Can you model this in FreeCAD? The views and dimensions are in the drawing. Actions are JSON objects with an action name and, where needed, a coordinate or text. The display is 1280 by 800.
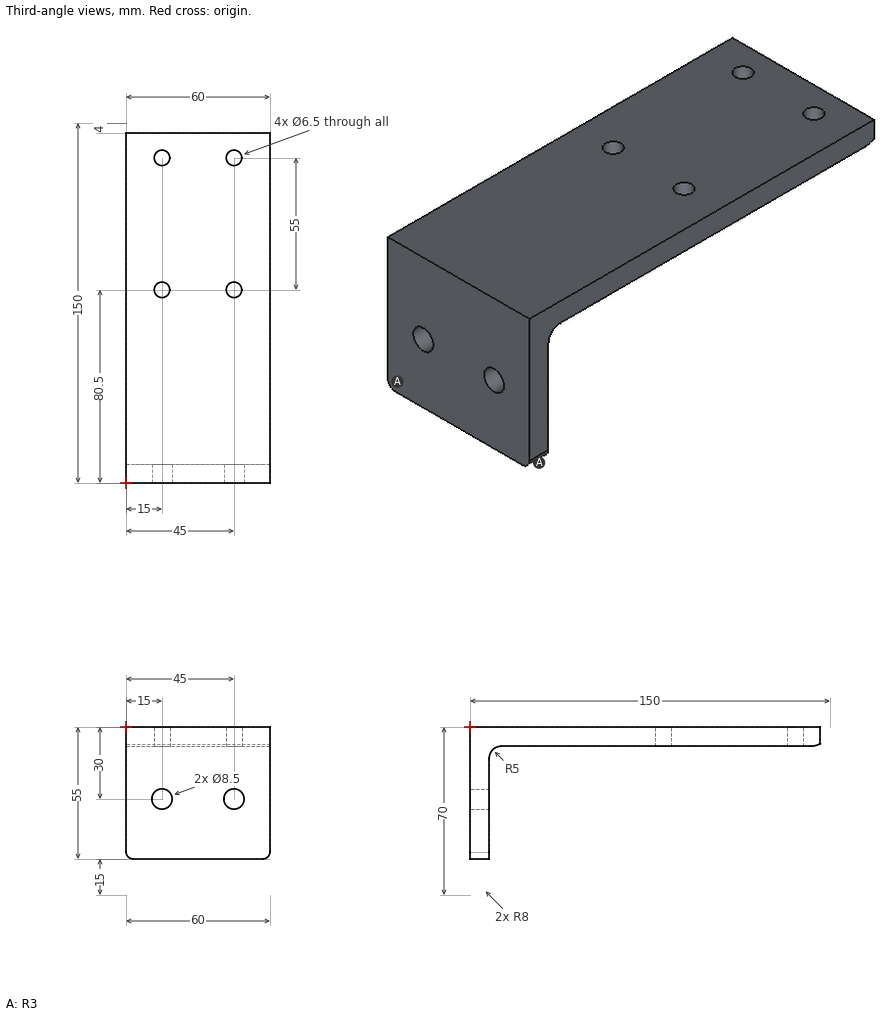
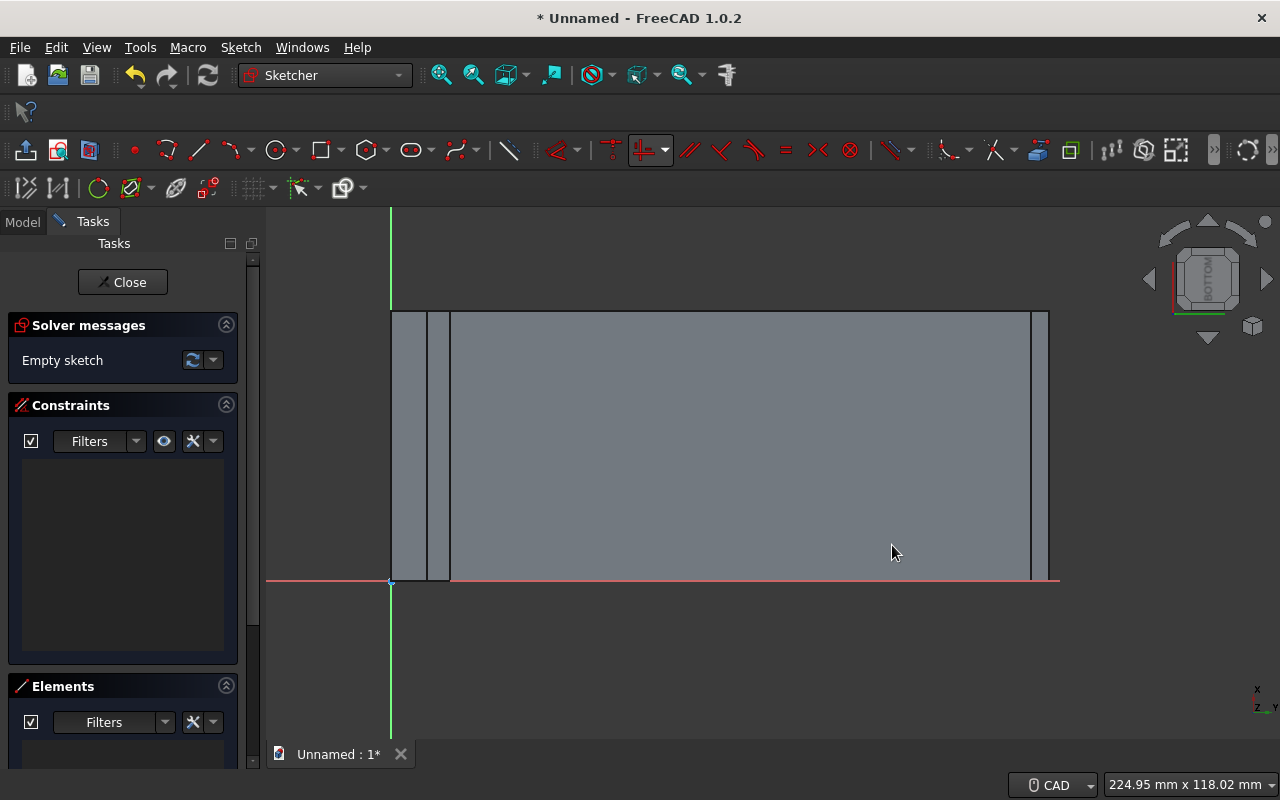
{"action": "left_click", "coordinate": [276, 150]}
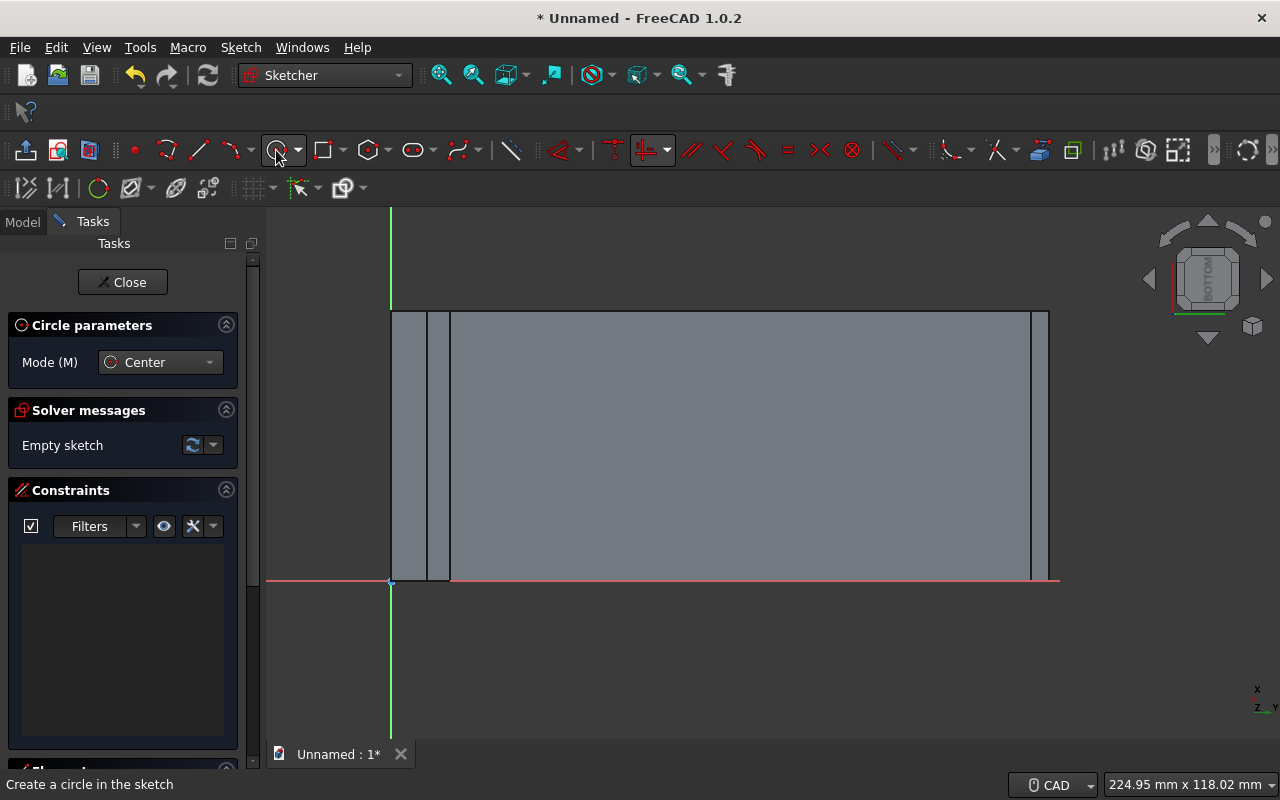
{"action": "scroll", "coordinate": [1002, 379], "scroll_direction": "up", "scroll_amount": 3}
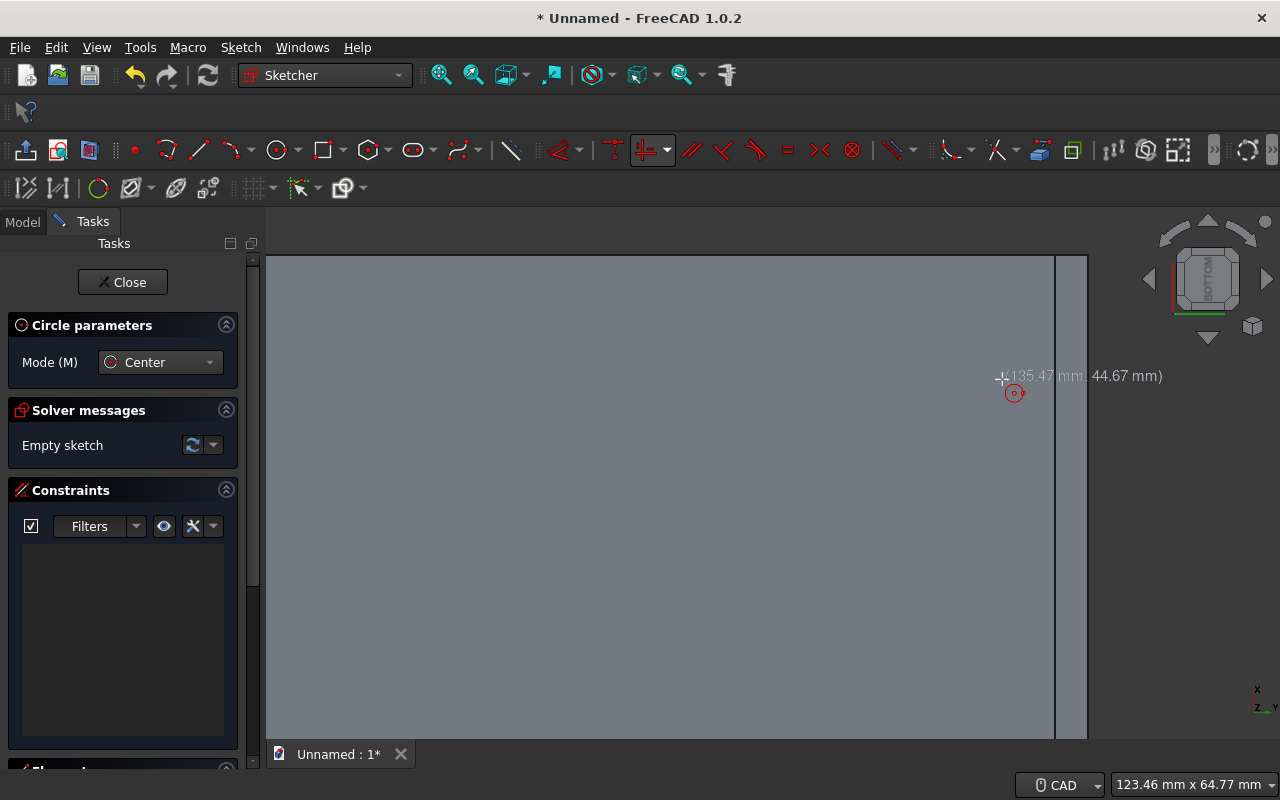
{"action": "left_click", "coordinate": [1002, 378]}
{"action": "left_click", "coordinate": [1021, 359]}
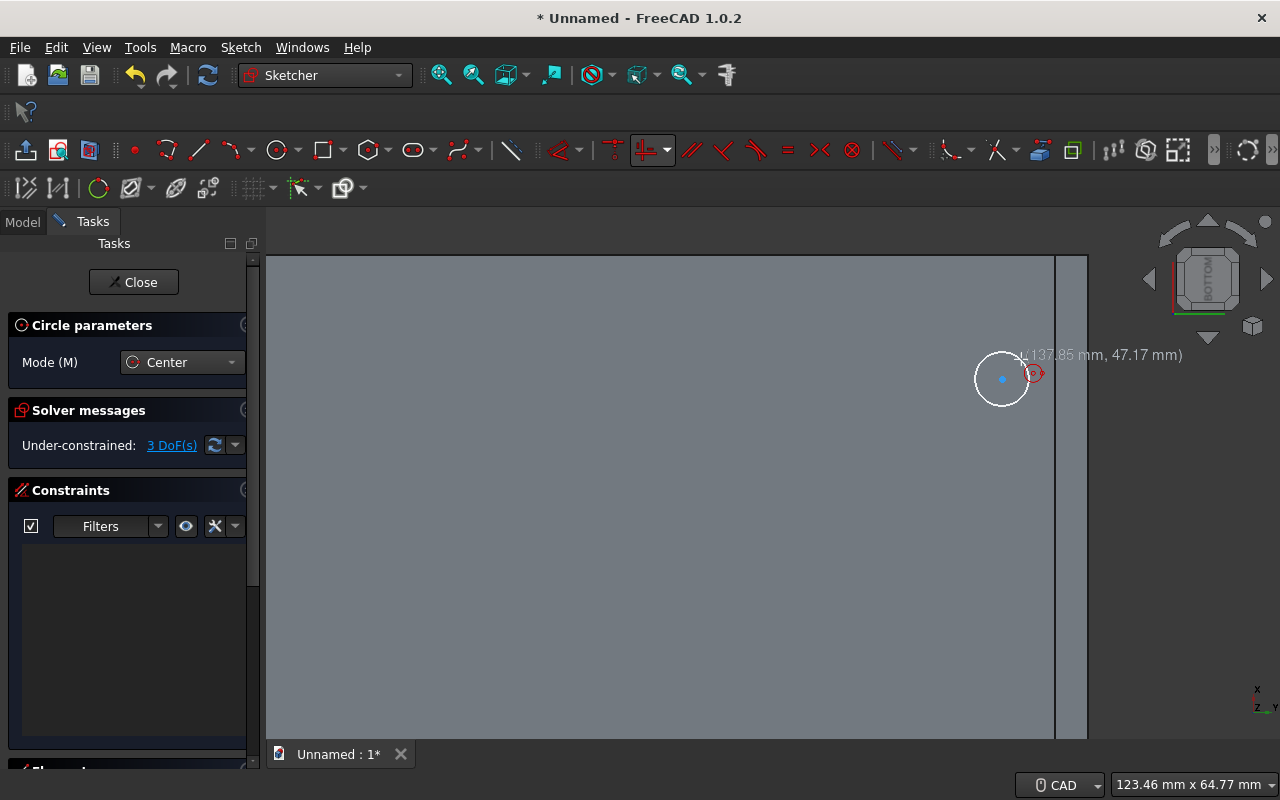
{"action": "left_click", "coordinate": [1002, 624]}
{"action": "left_click", "coordinate": [1021, 605]}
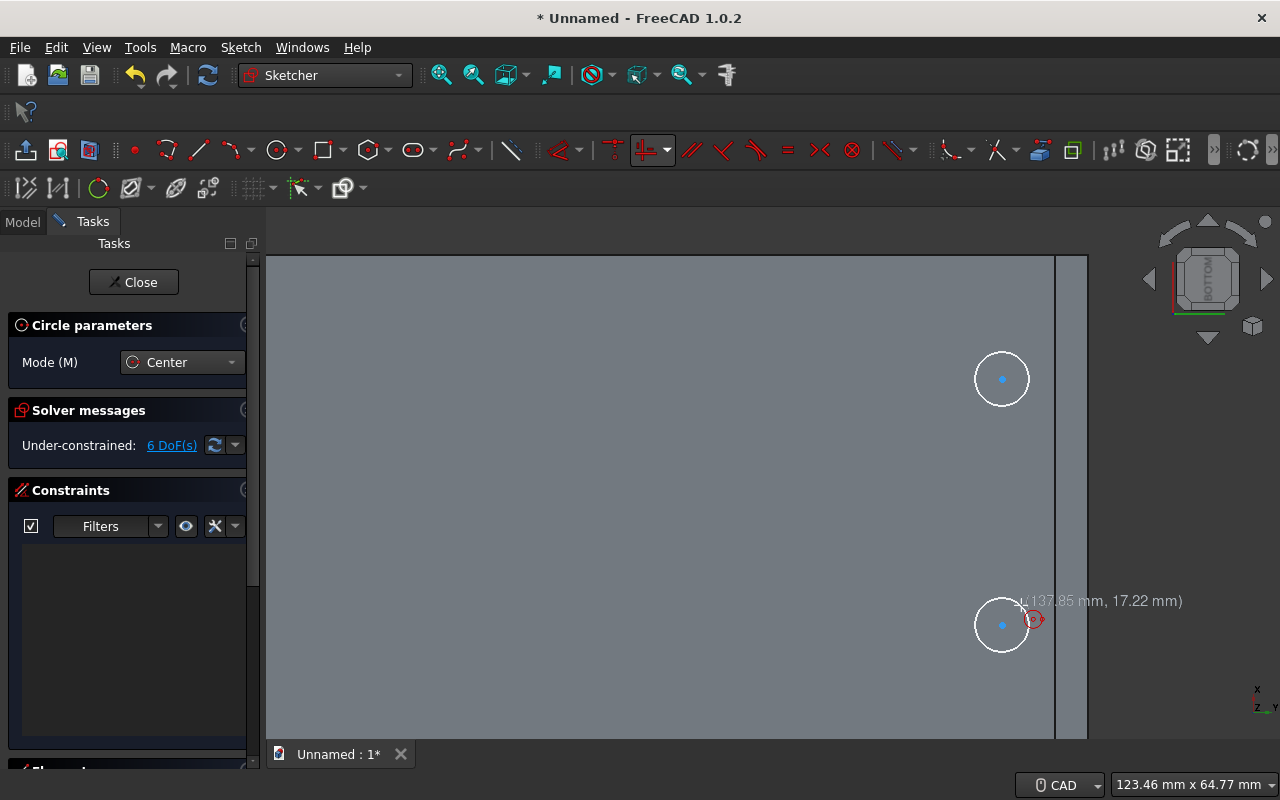
{"action": "left_click", "coordinate": [550, 378]}
{"action": "left_click", "coordinate": [569, 359]}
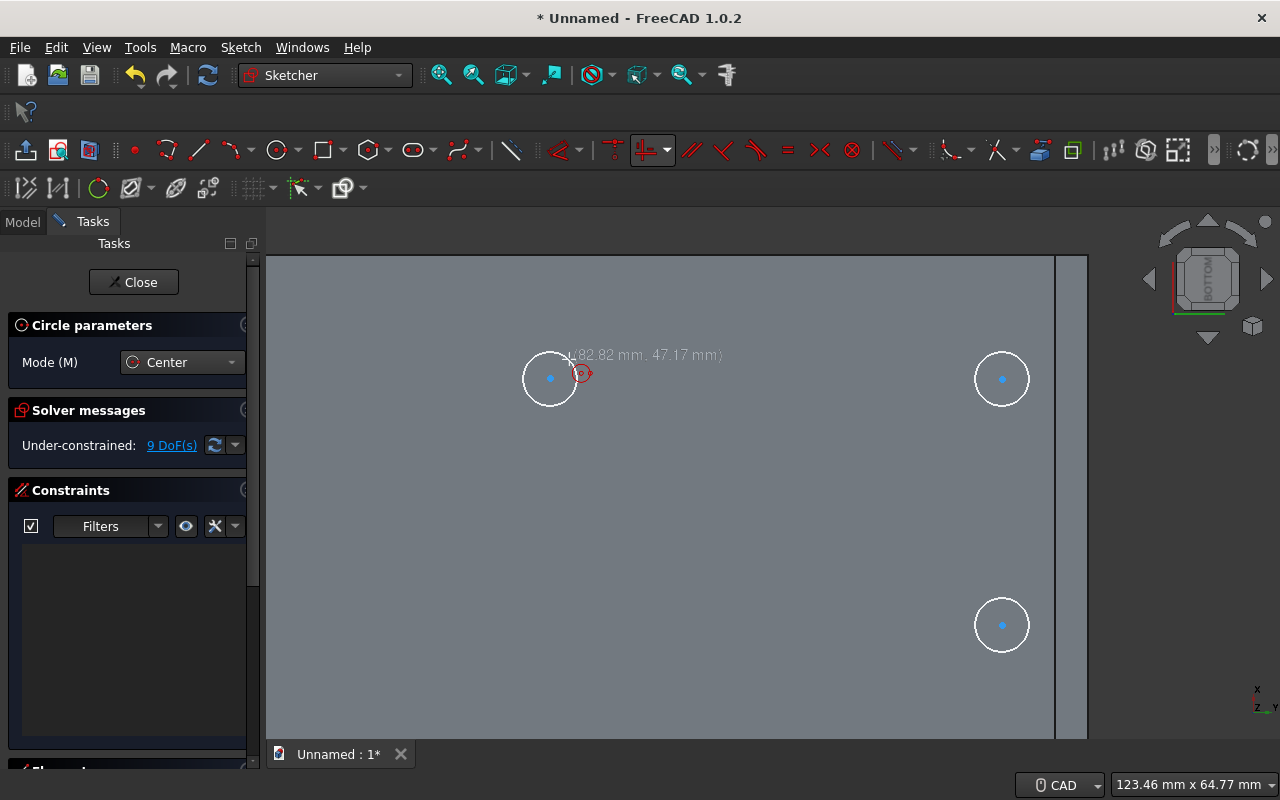
{"action": "left_click", "coordinate": [550, 624]}
{"action": "left_click", "coordinate": [569, 605]}
{"action": "key", "text": "Escape"}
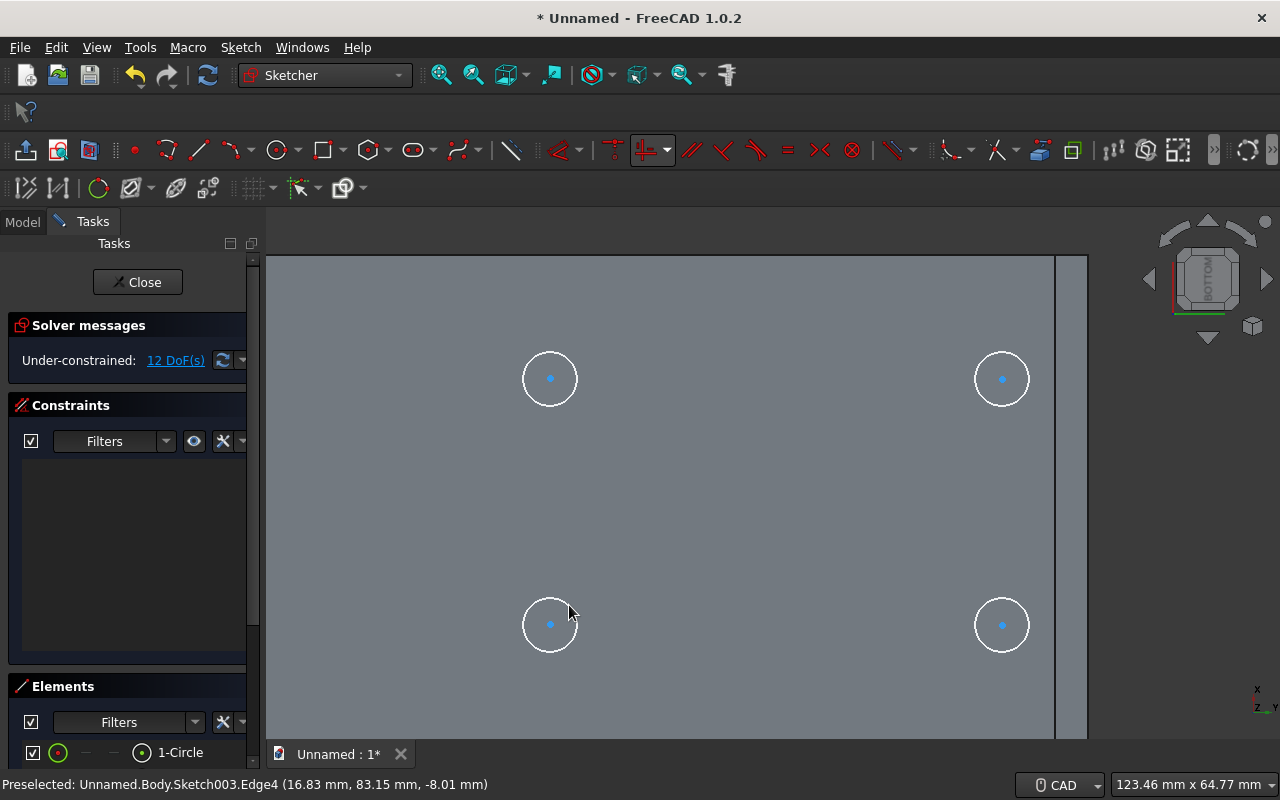
{"action": "left_click", "coordinate": [1021, 360]}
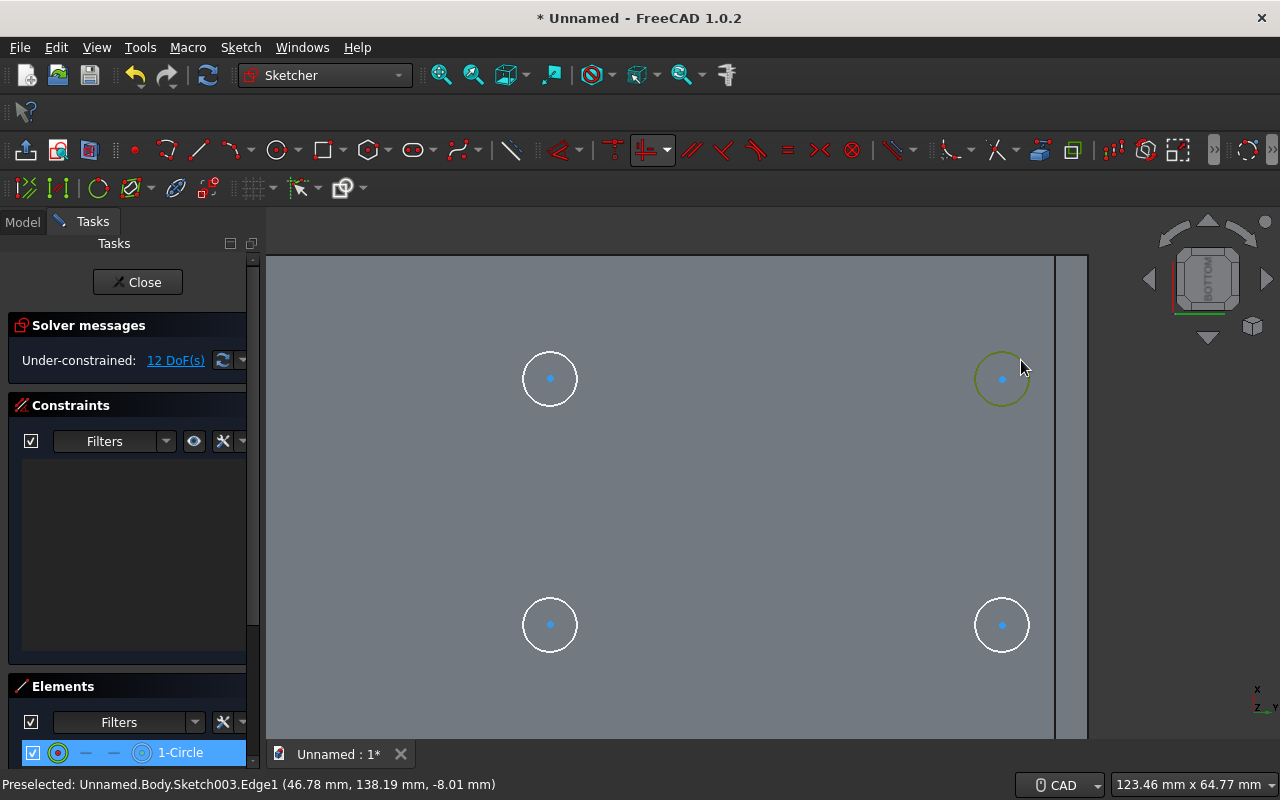
{"action": "left_click", "coordinate": [1021, 606]}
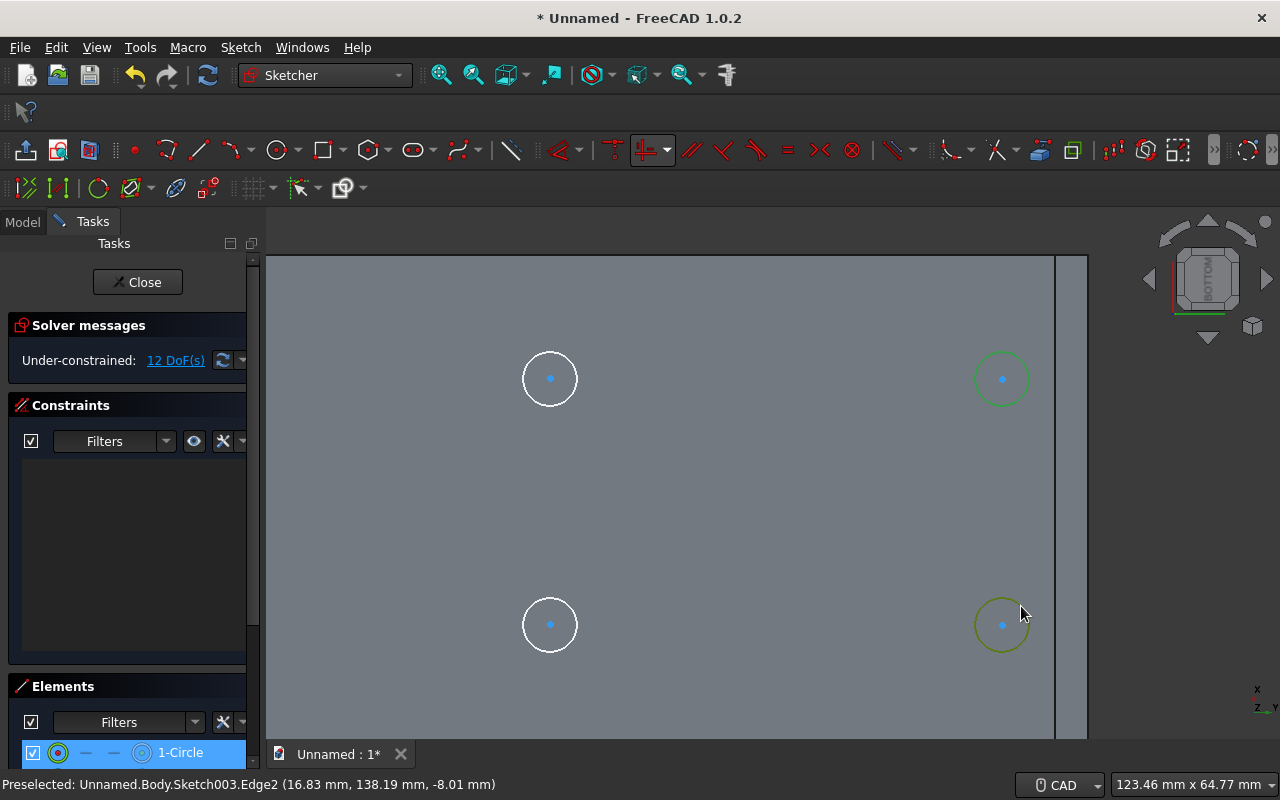
{"action": "left_click", "coordinate": [569, 360]}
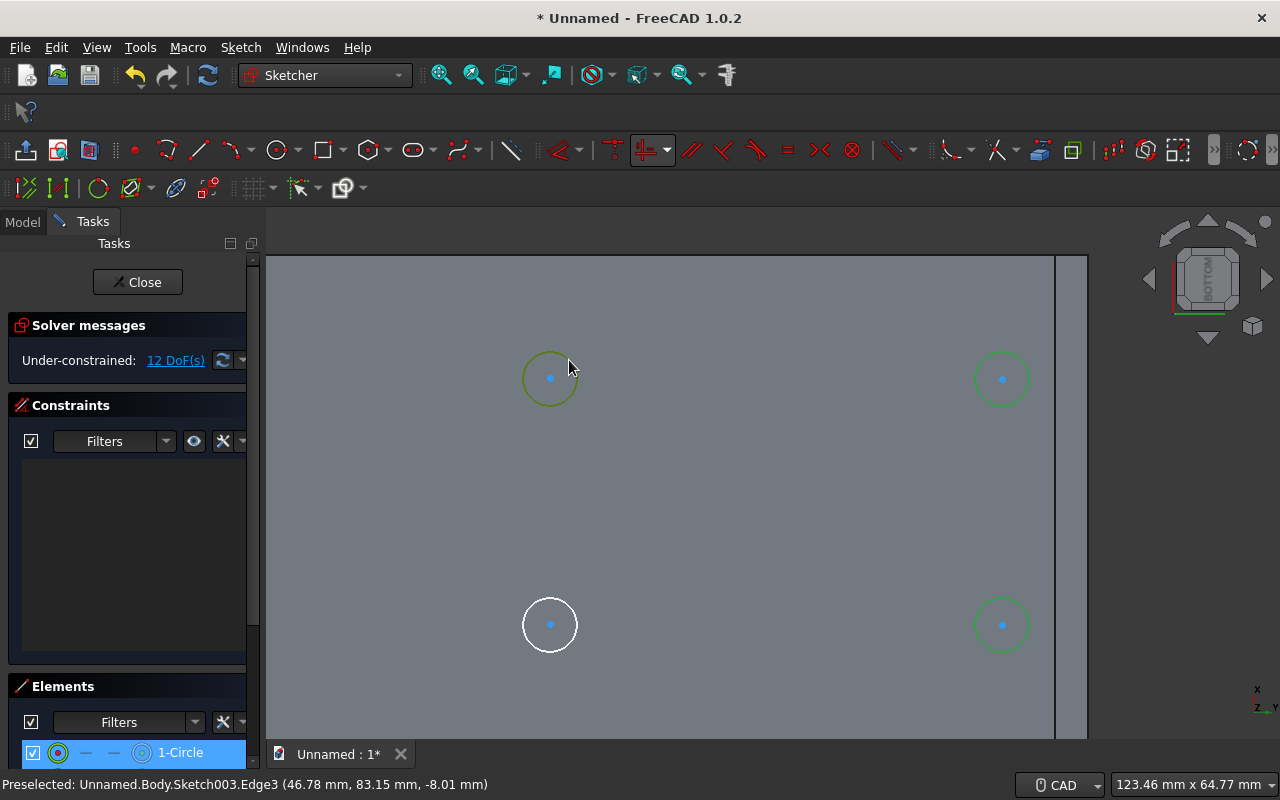
{"action": "left_click", "coordinate": [569, 606]}